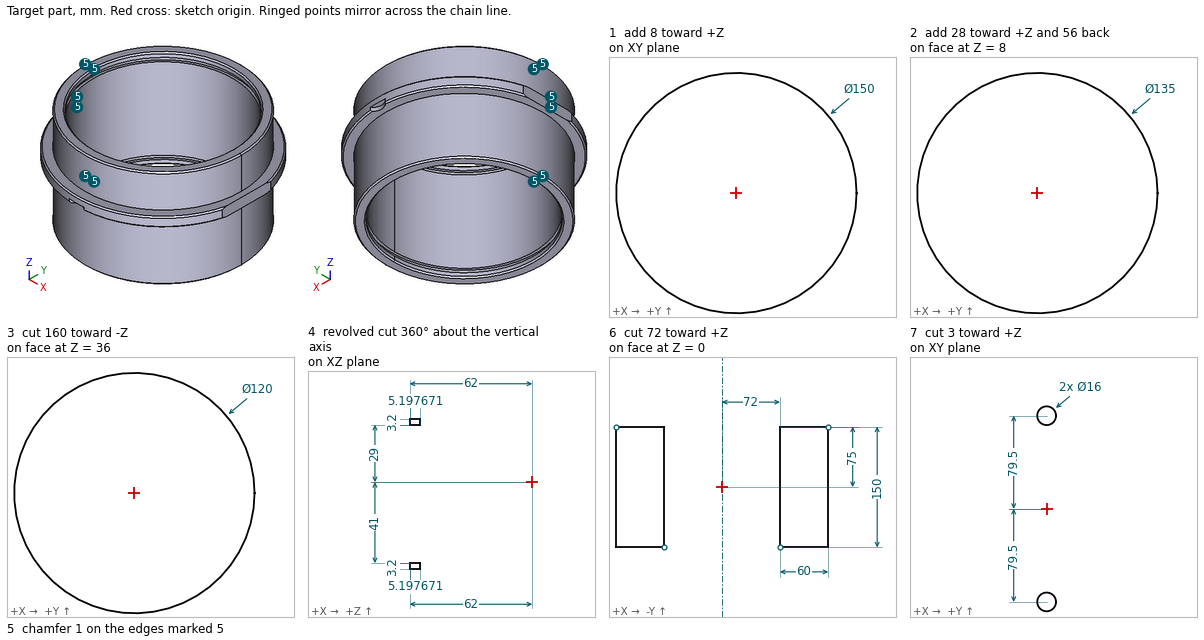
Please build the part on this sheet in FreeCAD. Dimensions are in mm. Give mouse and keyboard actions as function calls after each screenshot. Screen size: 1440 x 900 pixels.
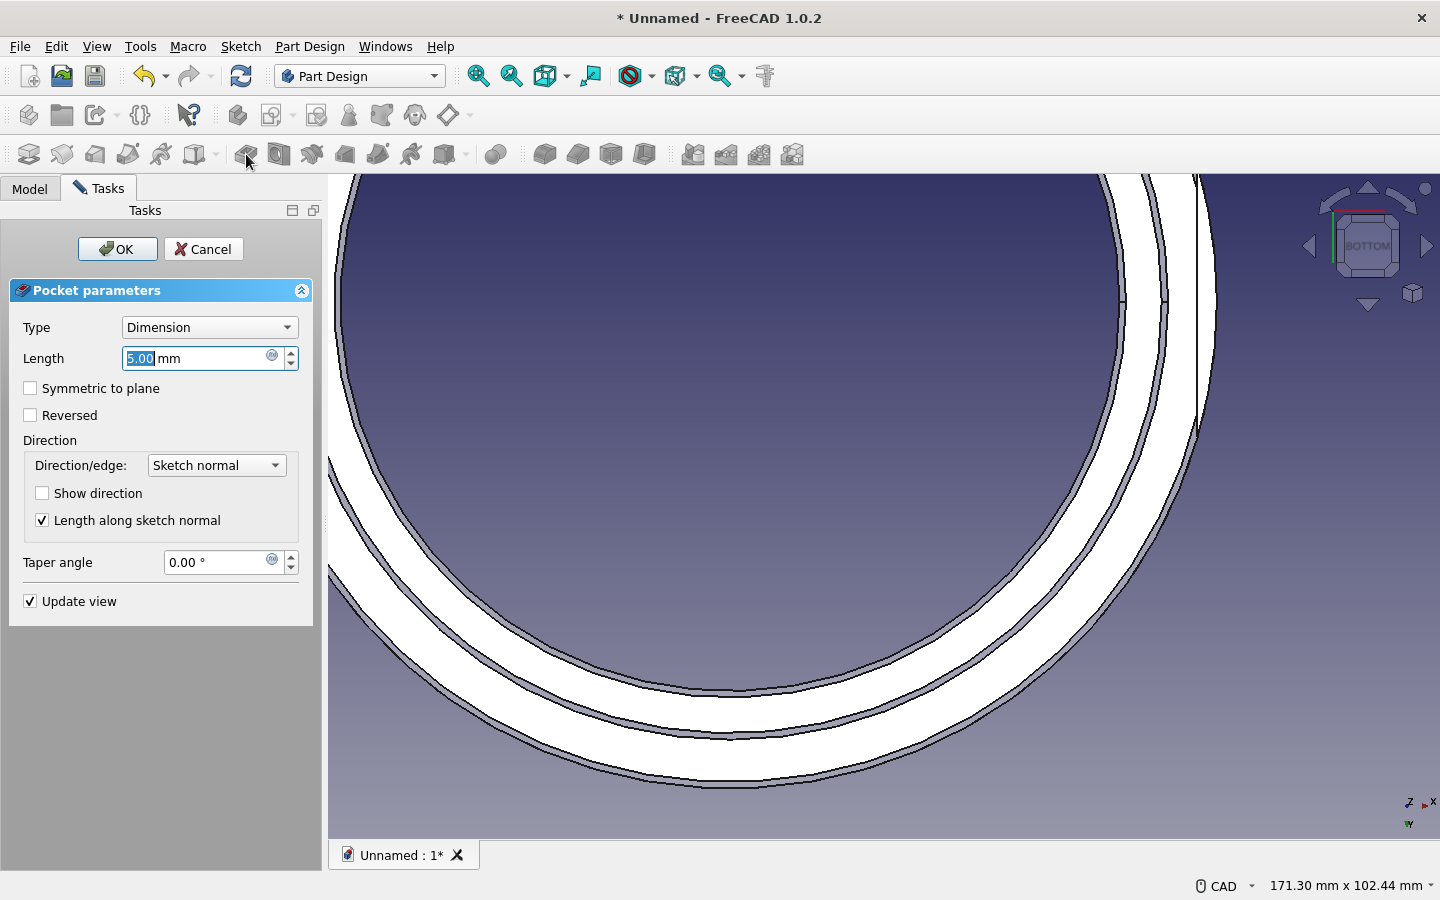
text(72)
key(Tab)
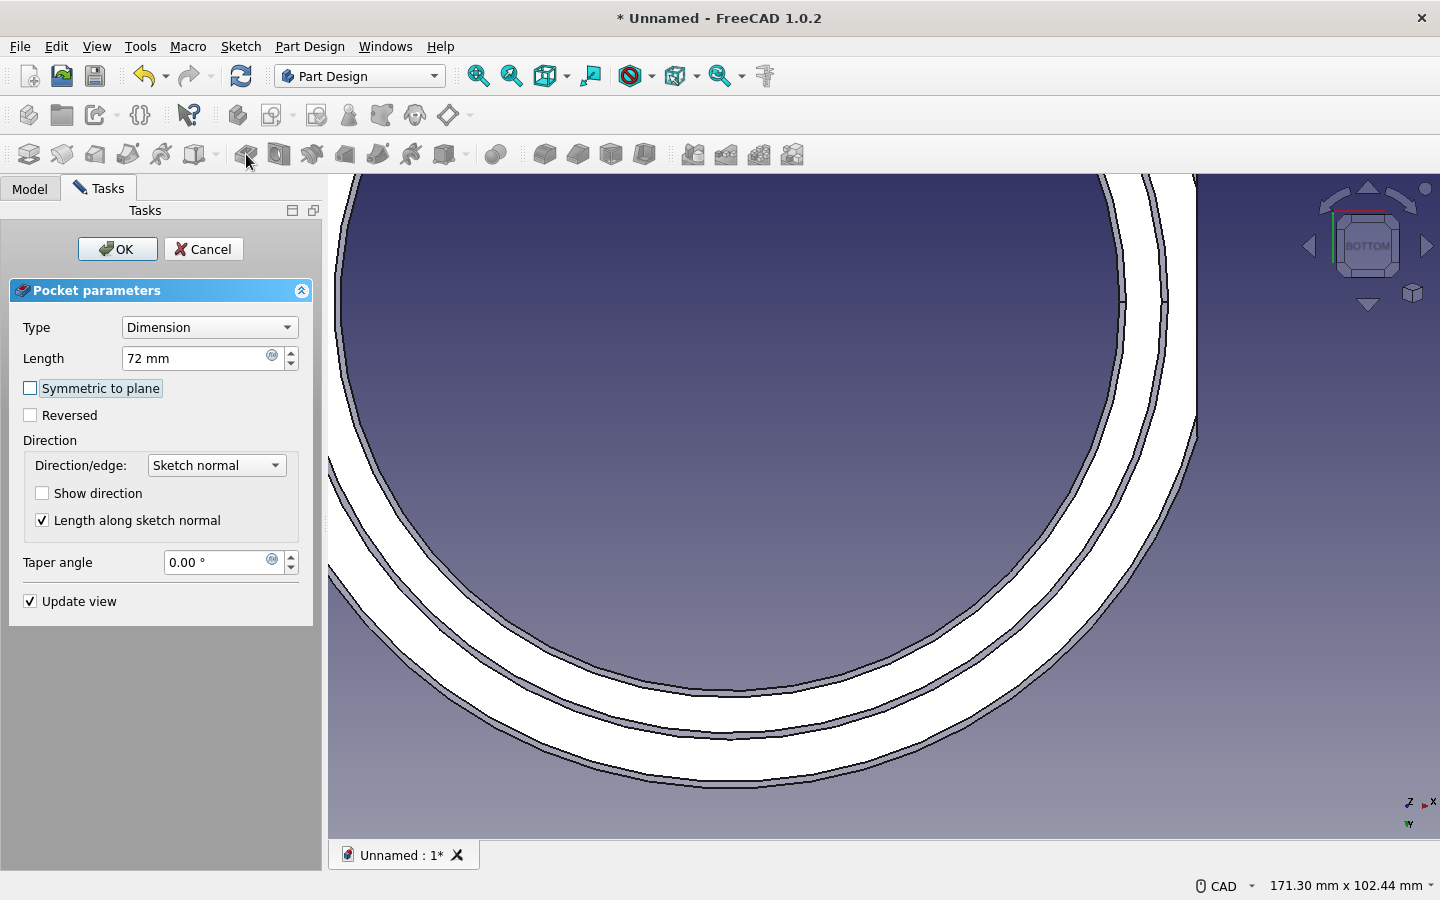
click(118, 249)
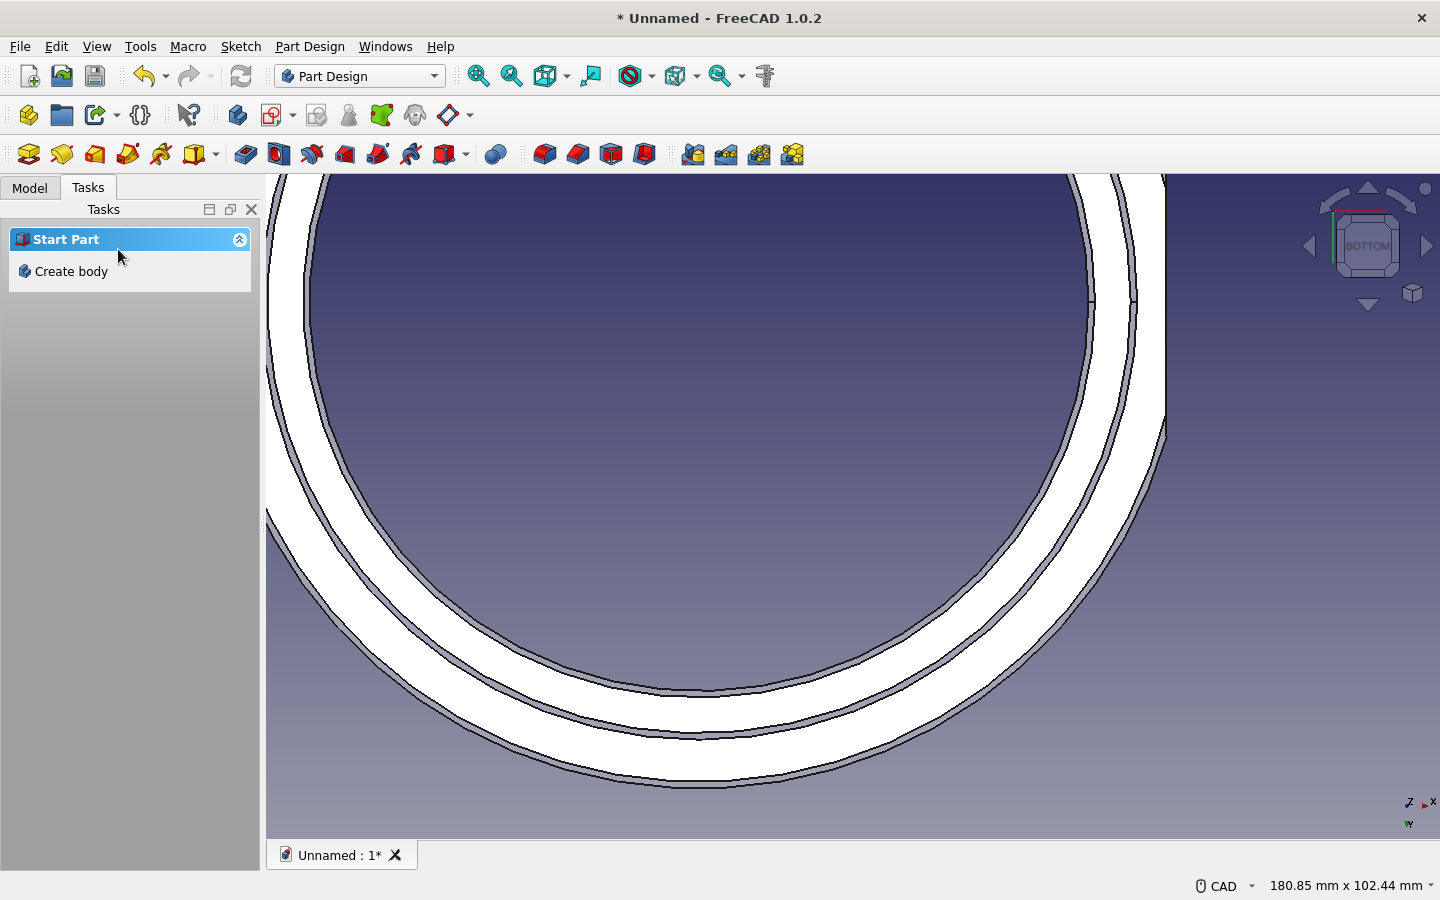
key(v)
key(f)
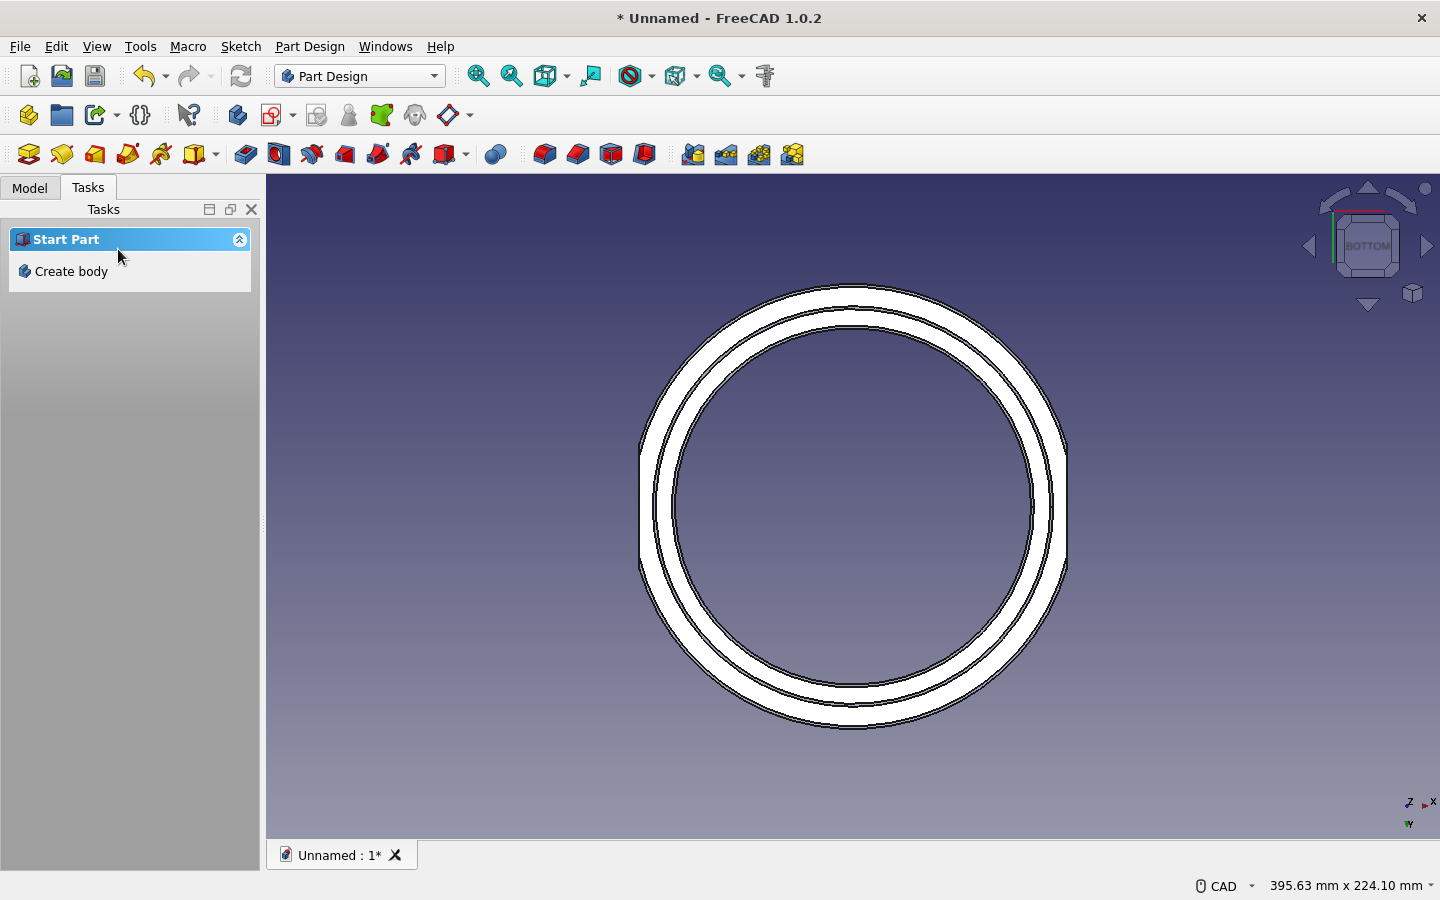
click(270, 116)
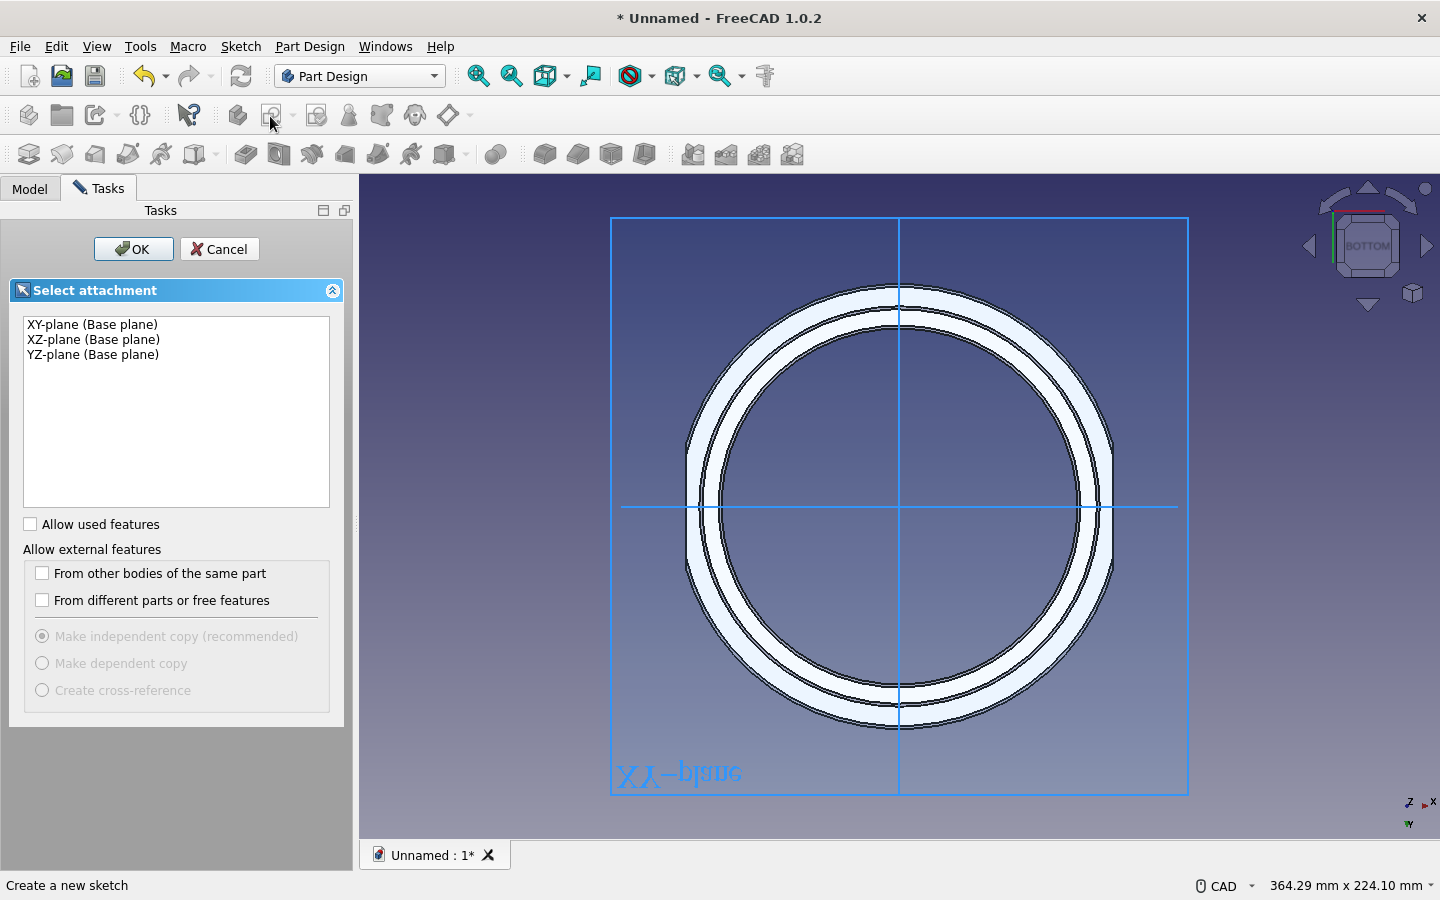
click(84, 324)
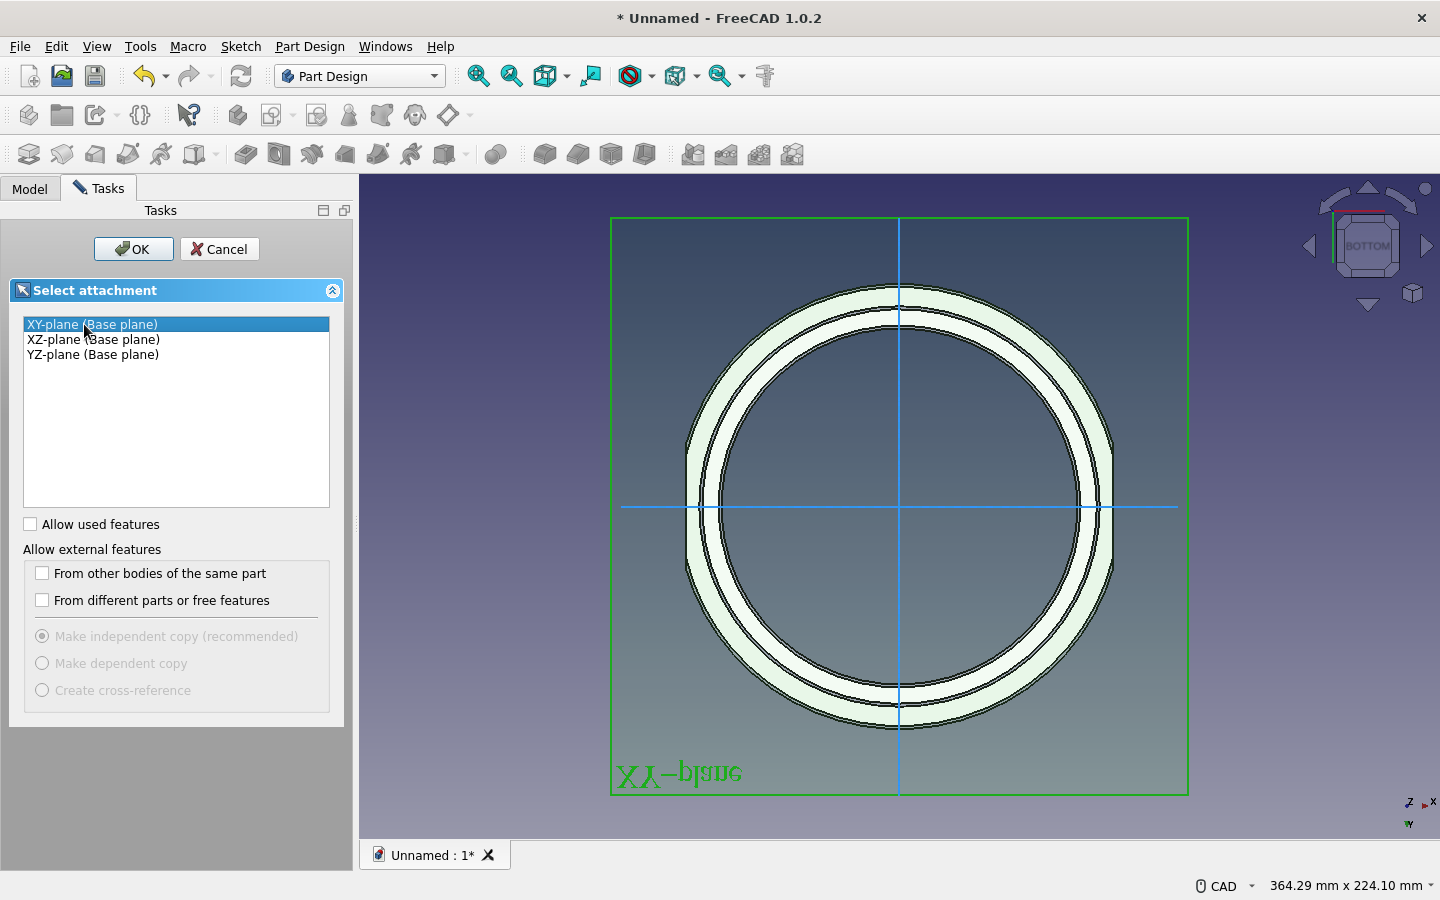
click(134, 249)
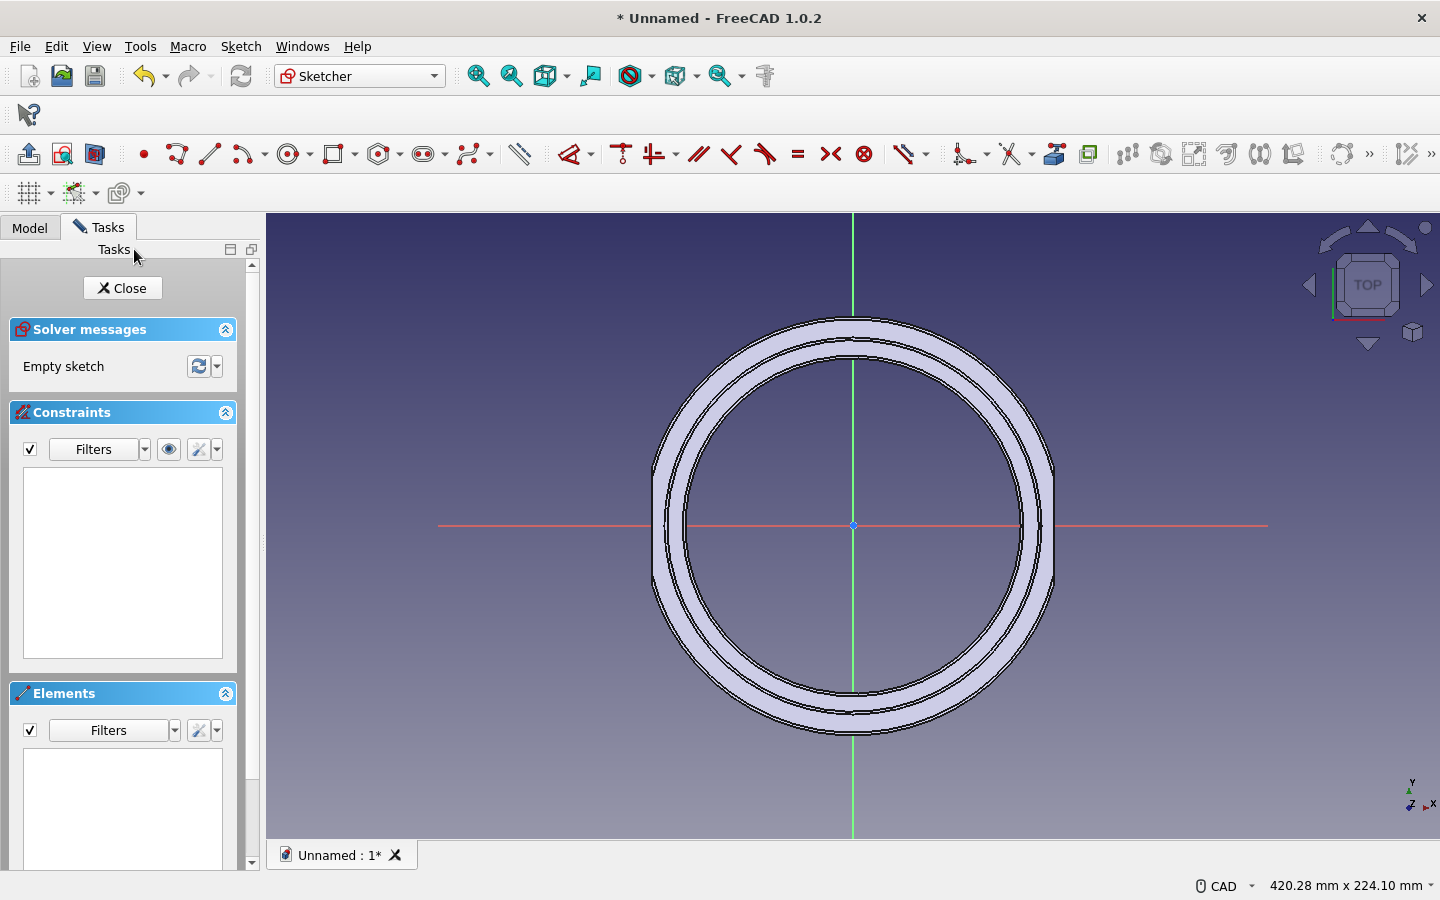
key(q)
key(s)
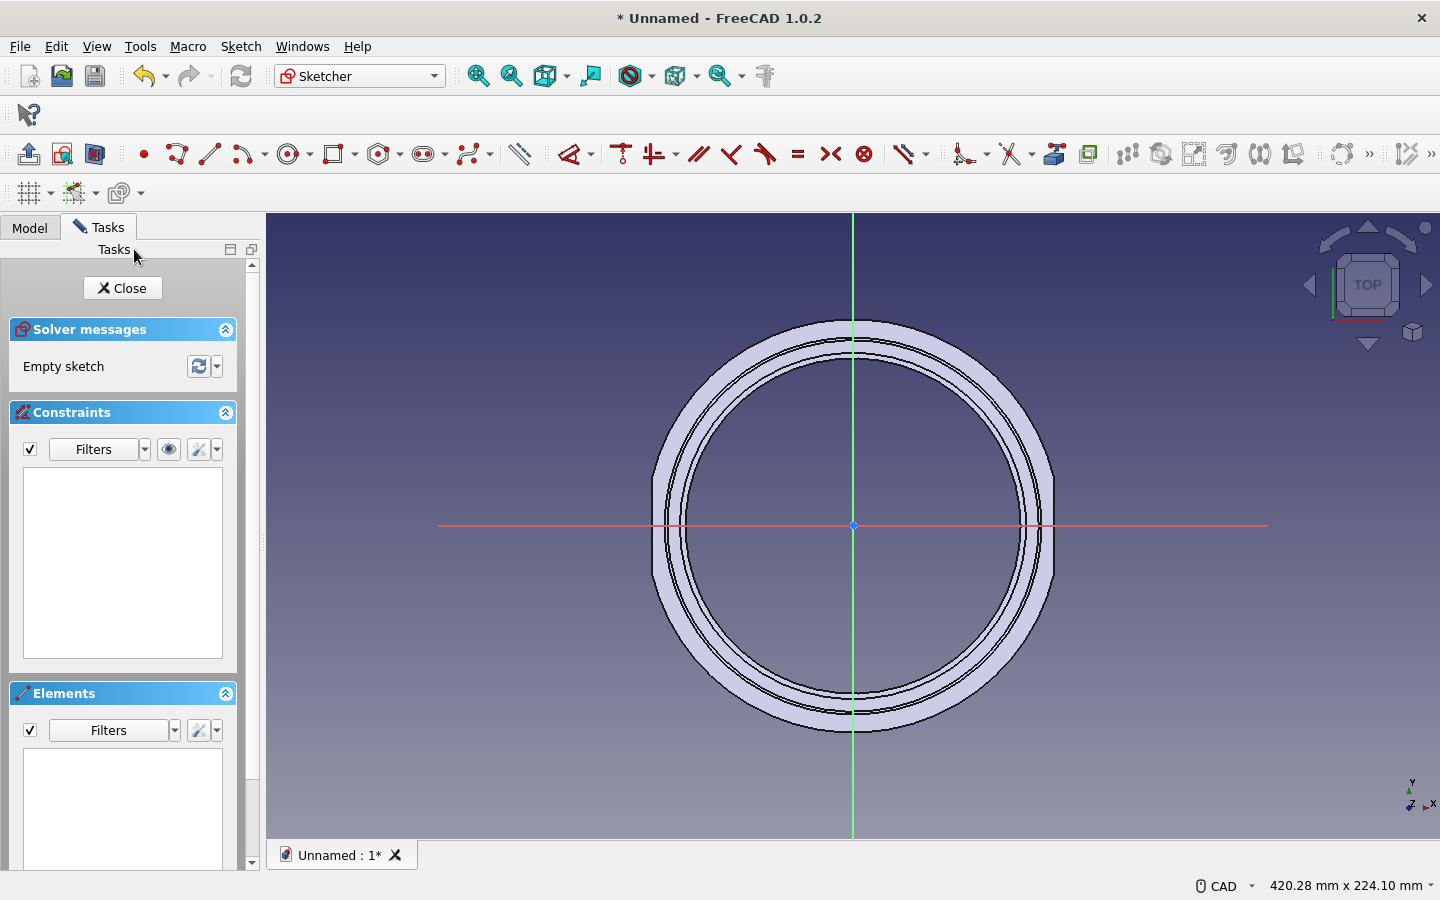
click(288, 154)